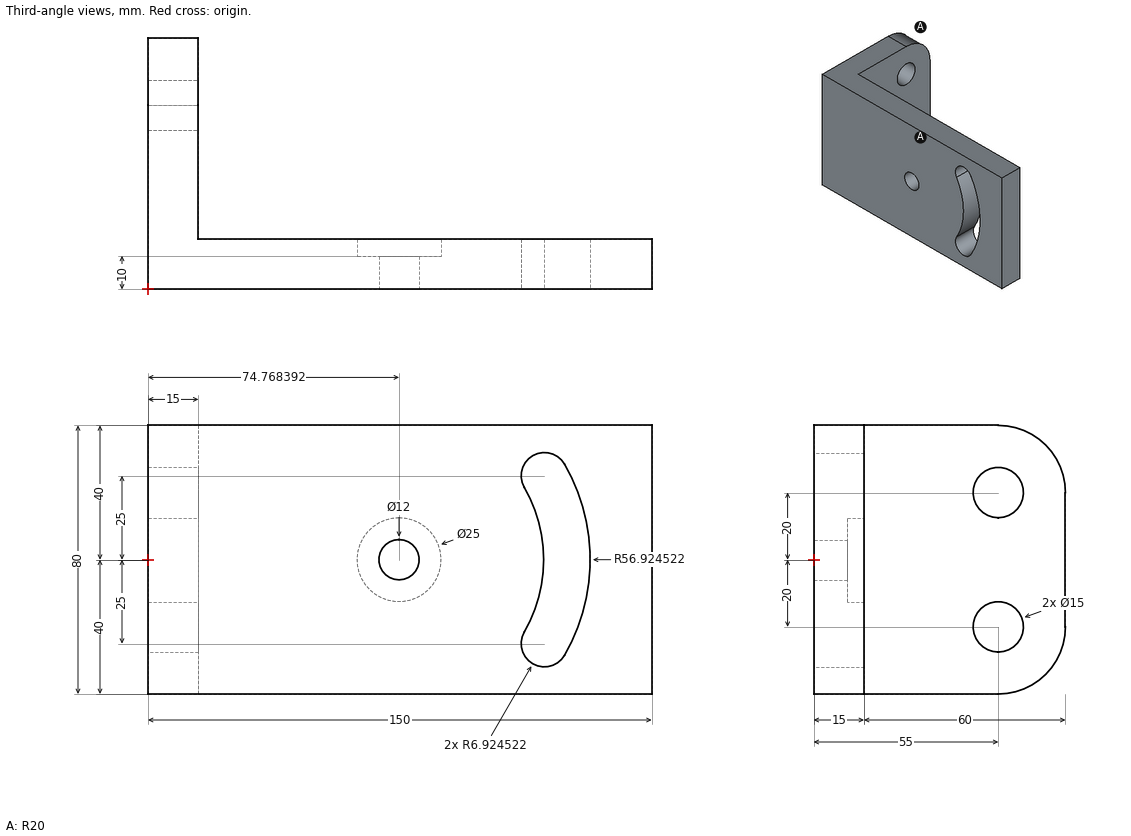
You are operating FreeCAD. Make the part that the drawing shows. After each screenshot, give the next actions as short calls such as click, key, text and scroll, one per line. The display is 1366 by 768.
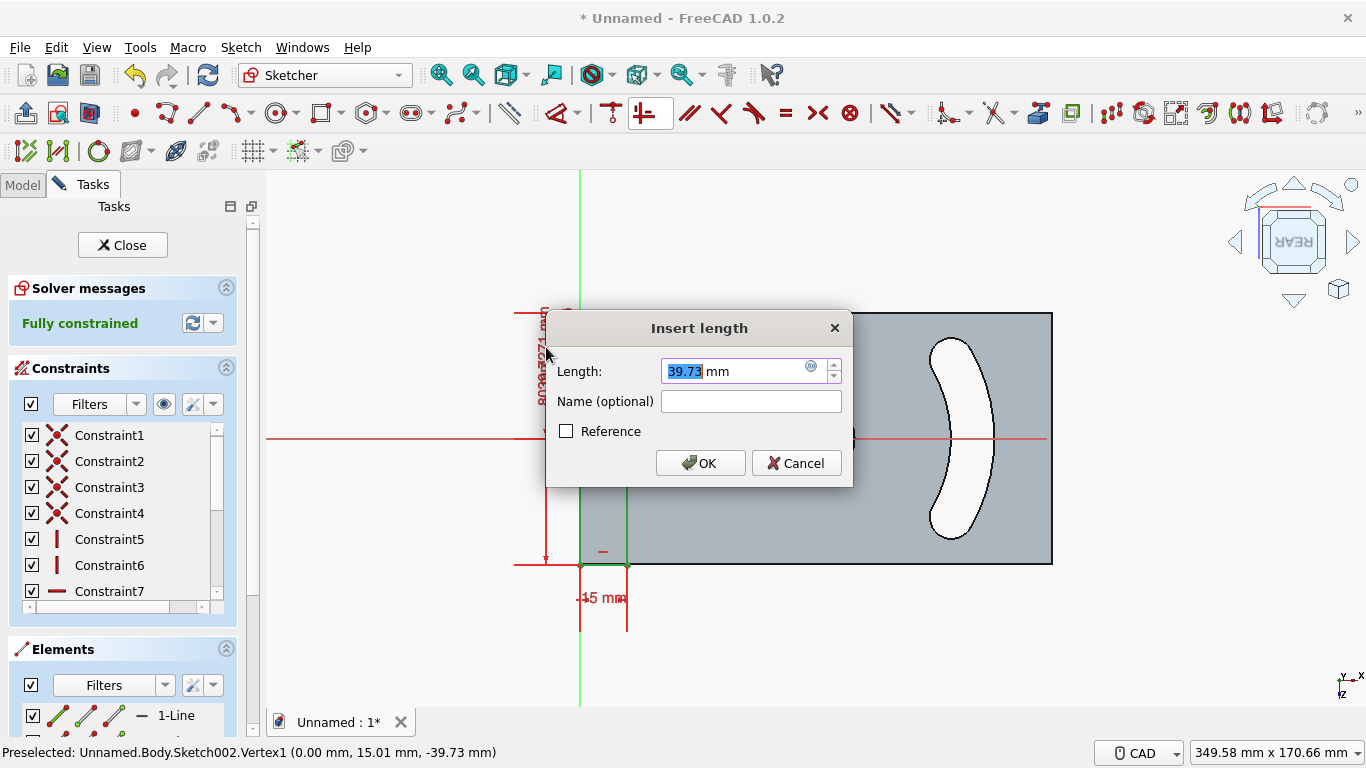
text(40)
key(Return)
key(Escape)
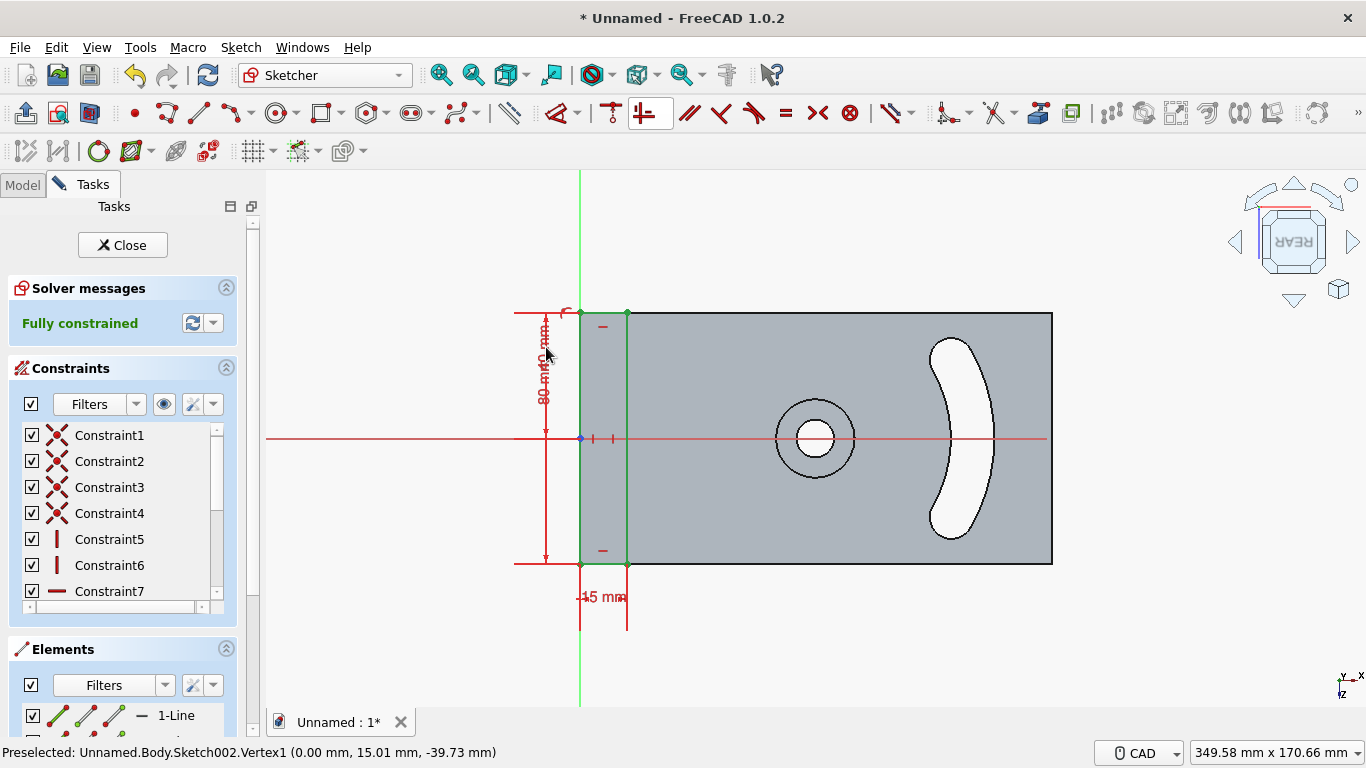
click(123, 245)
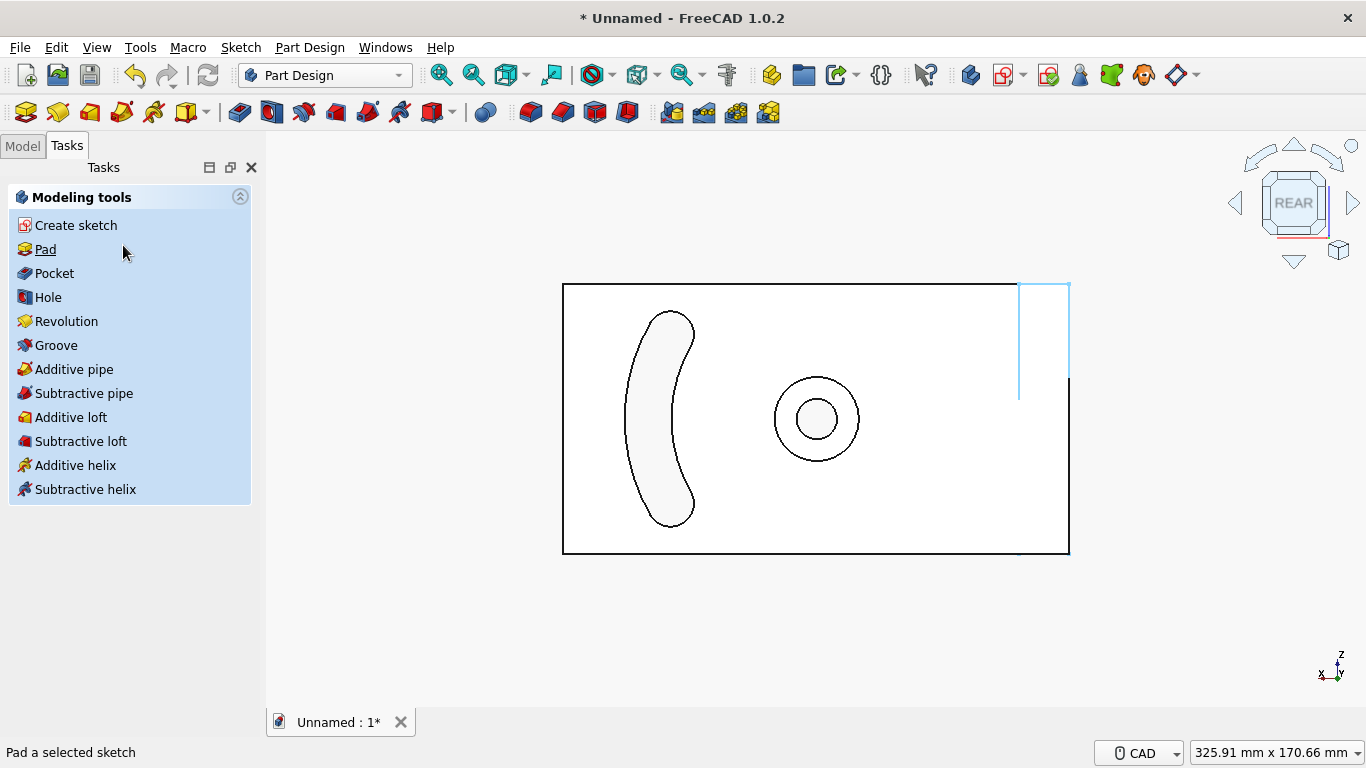
click(26, 112)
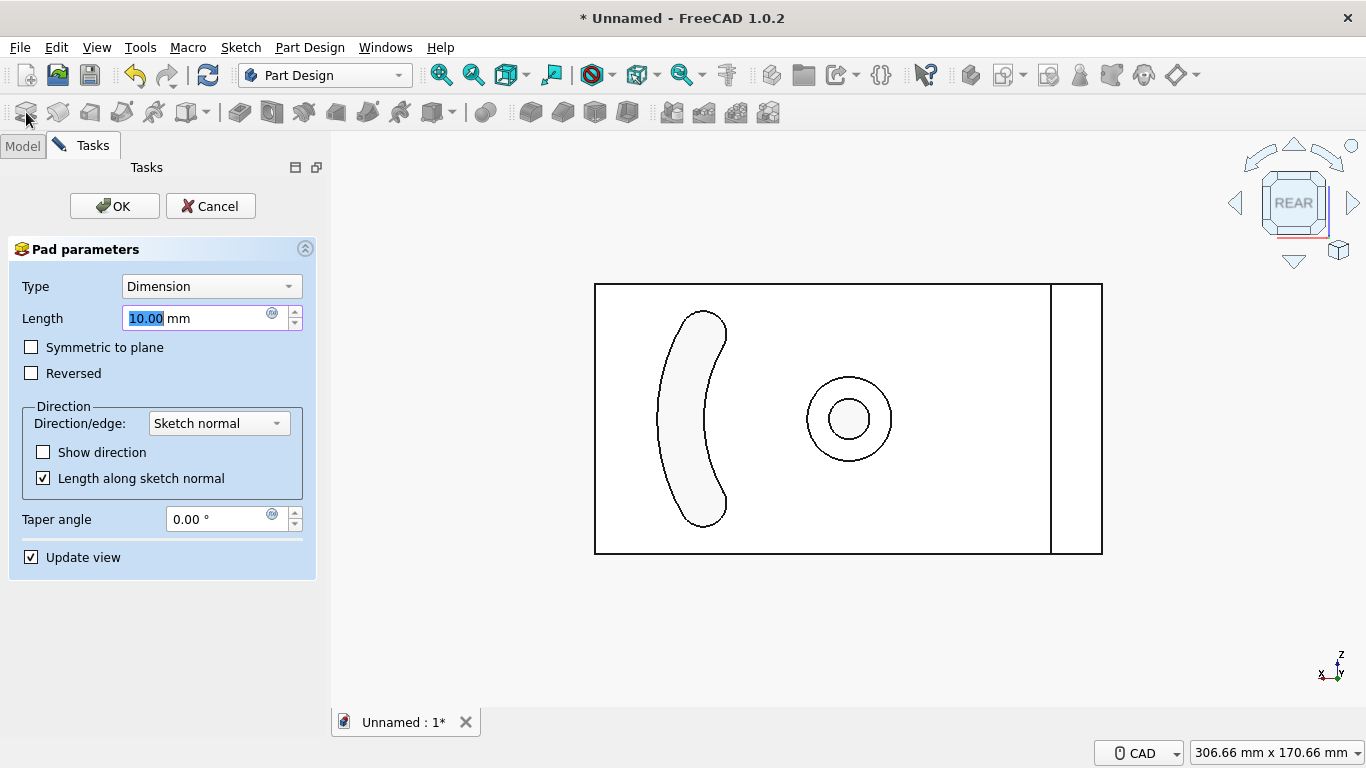
text(60)
key(Tab)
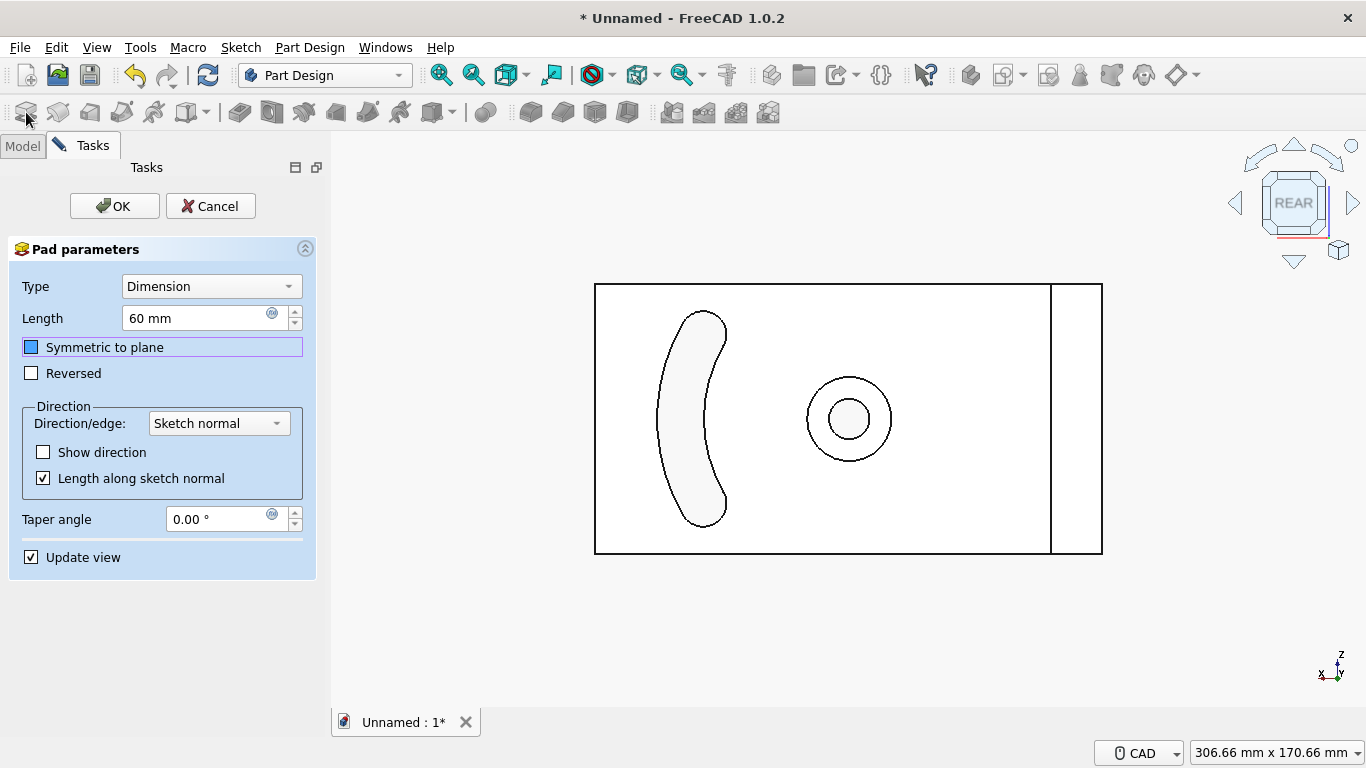
click(115, 206)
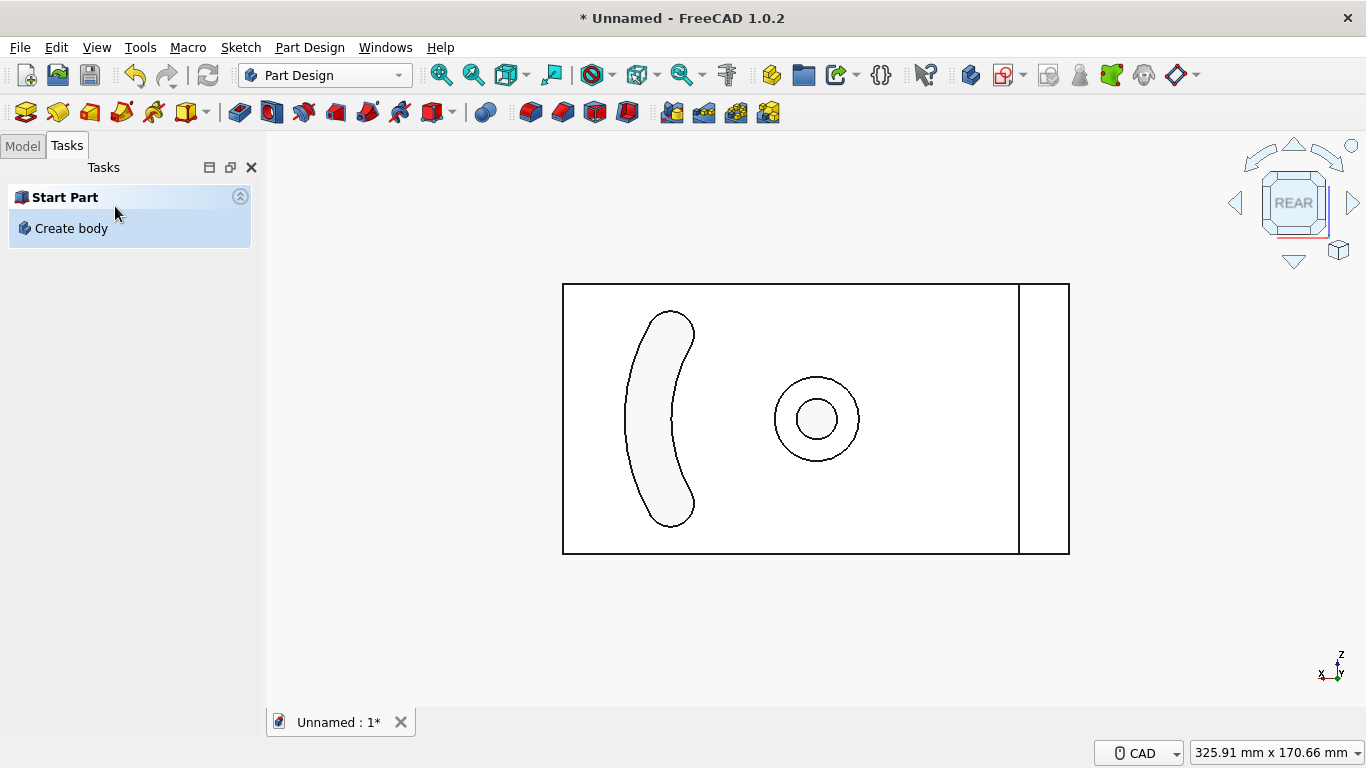
click(1044, 553)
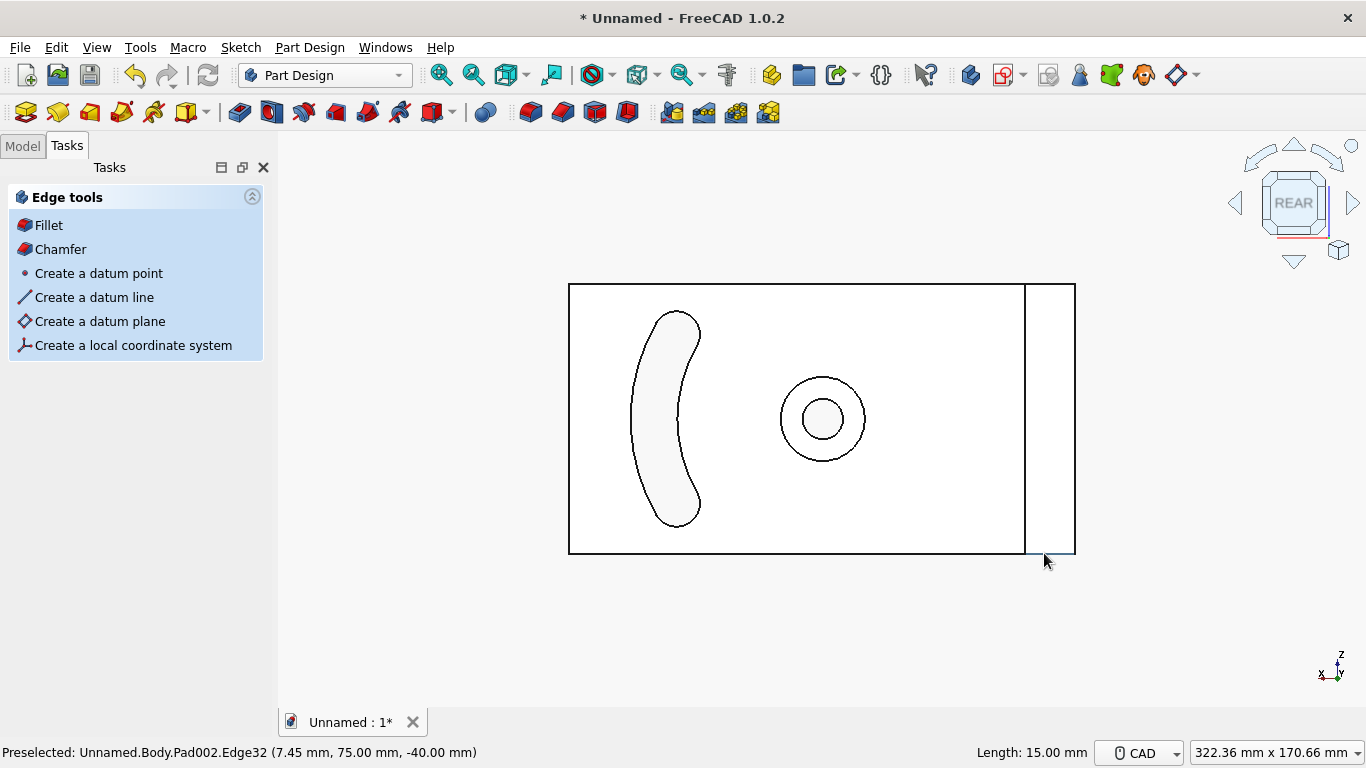
key(0)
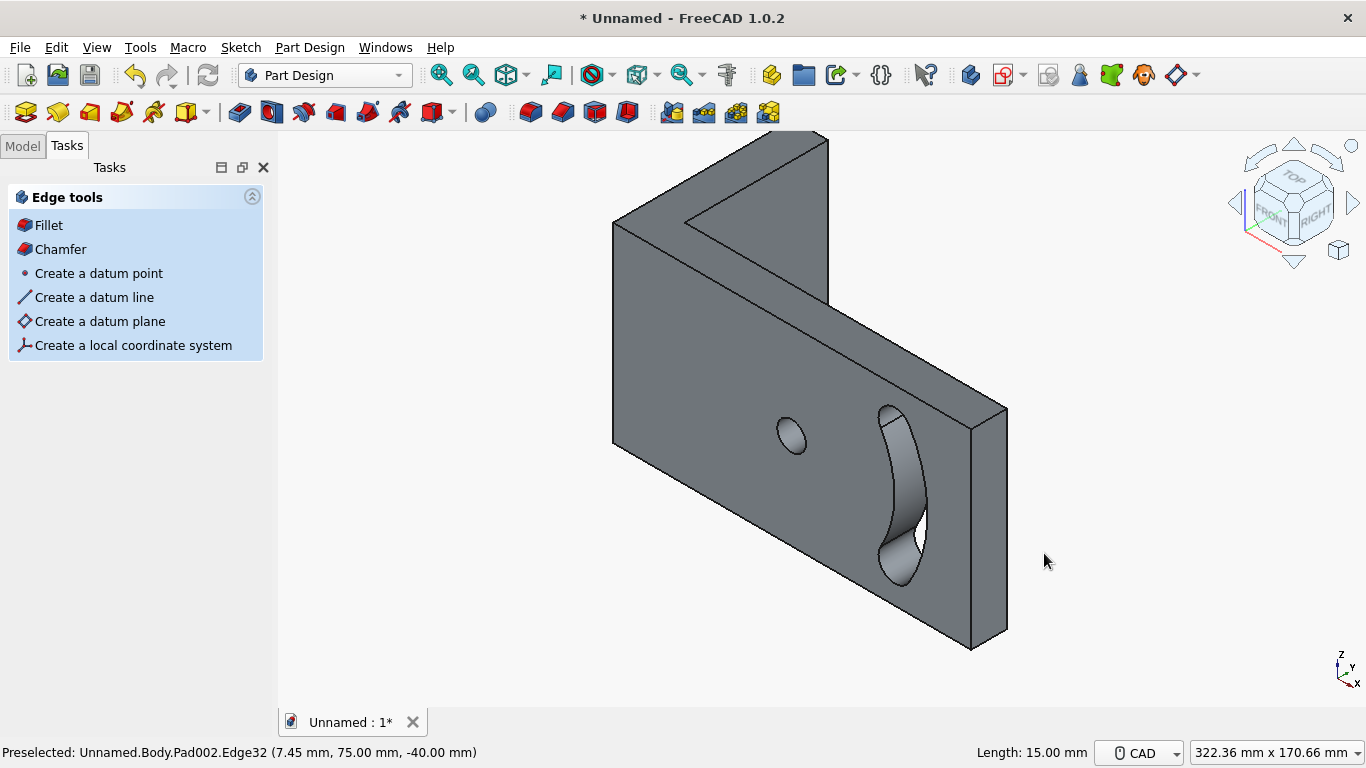
click(442, 76)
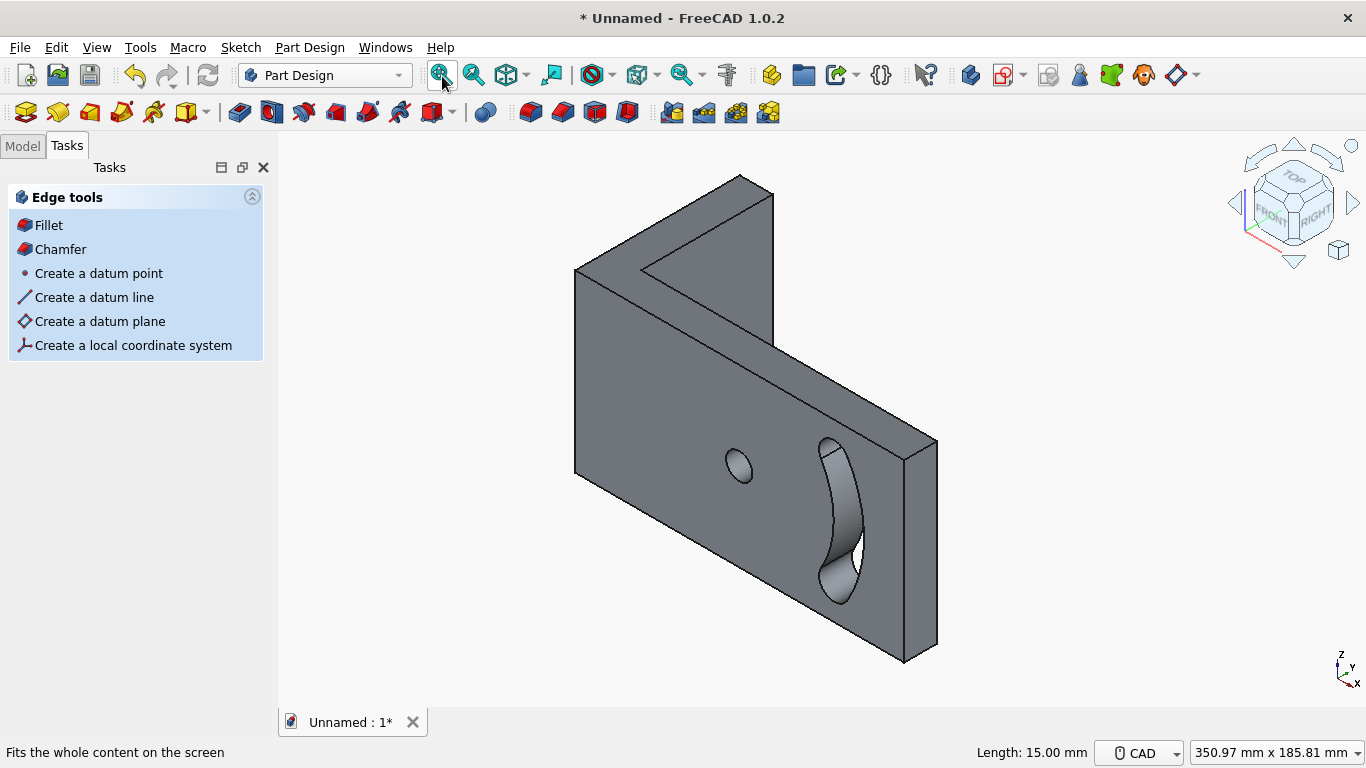
key(2)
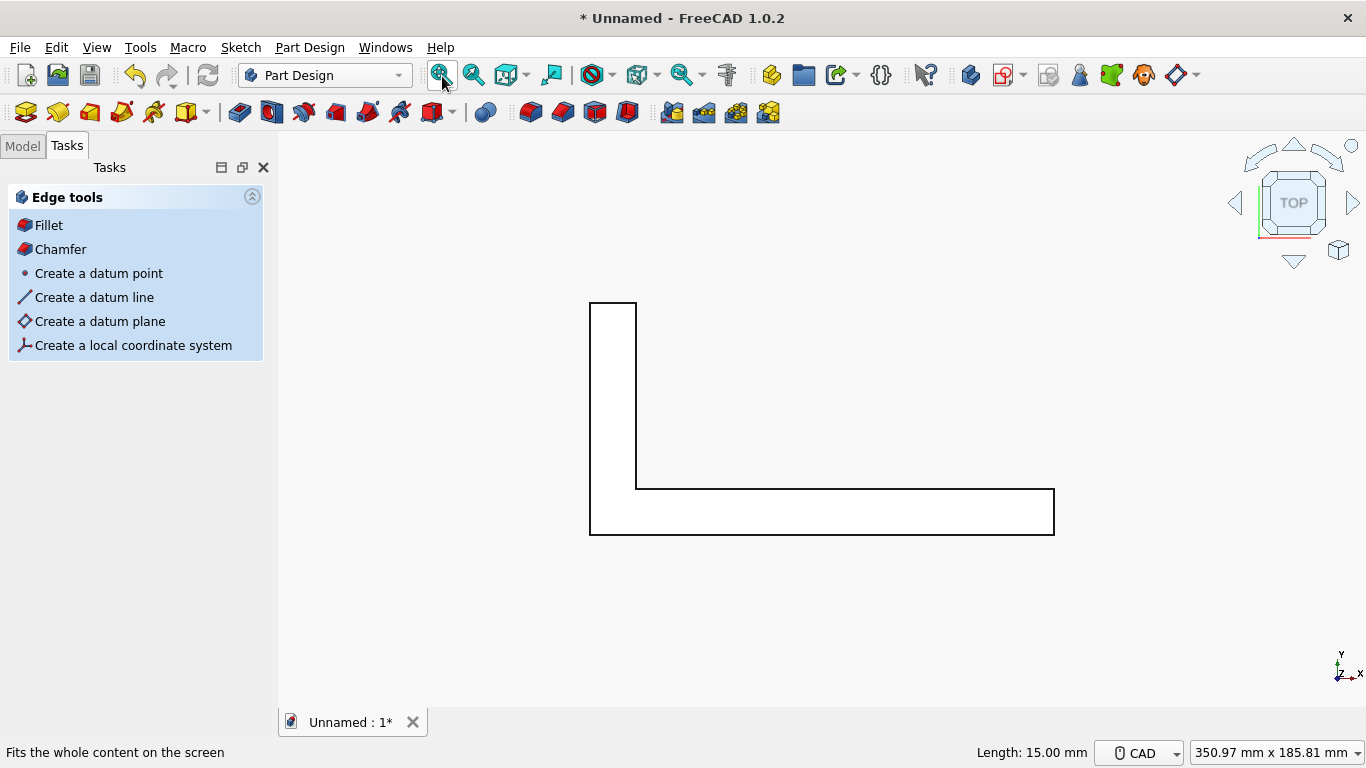
click(442, 76)